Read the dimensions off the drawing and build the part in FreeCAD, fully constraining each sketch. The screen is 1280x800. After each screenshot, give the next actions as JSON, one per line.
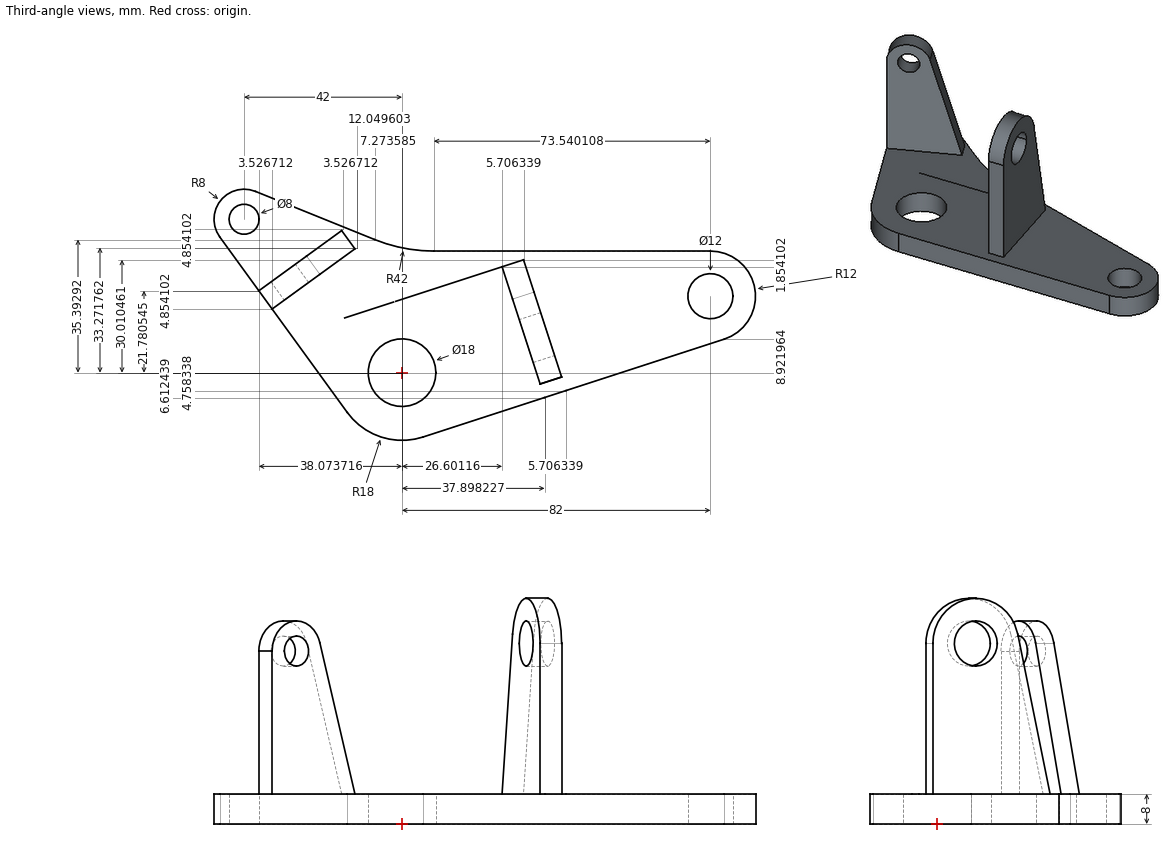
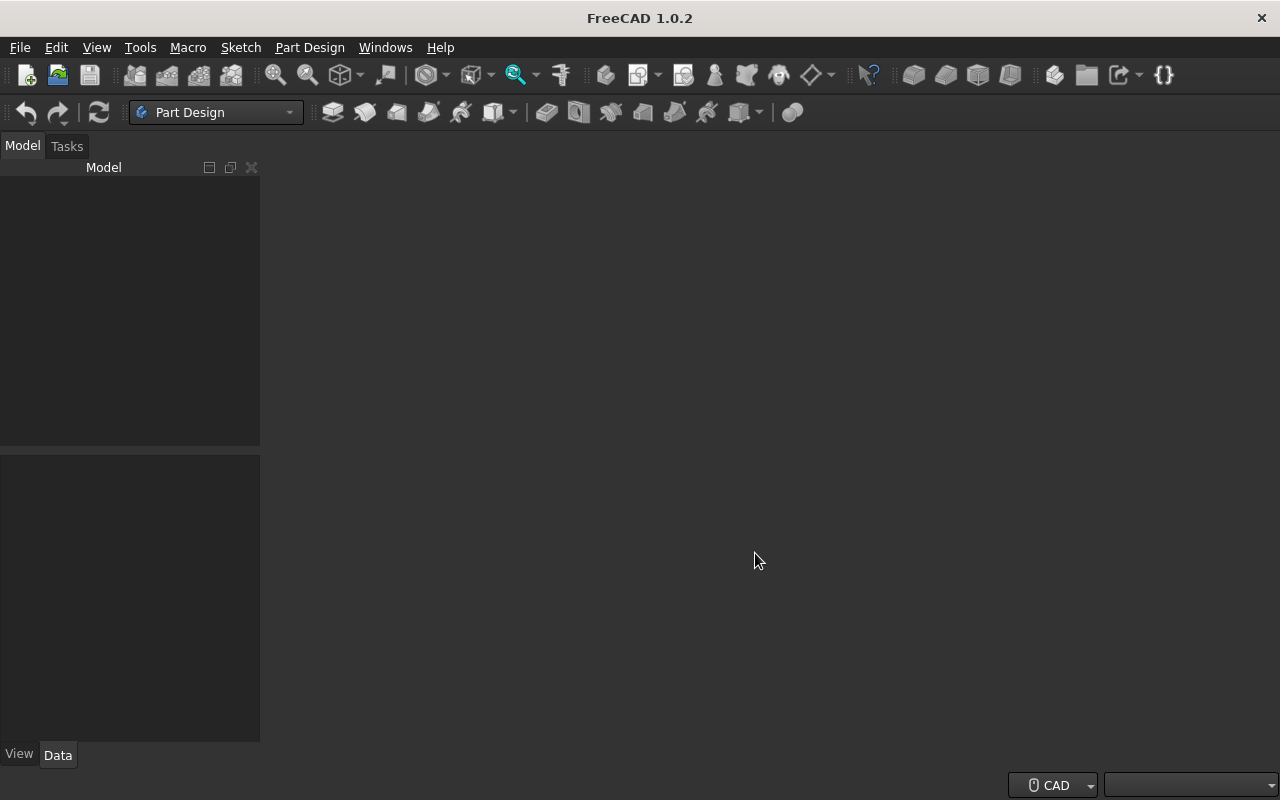
{"action": "left_click", "coordinate": [26, 76]}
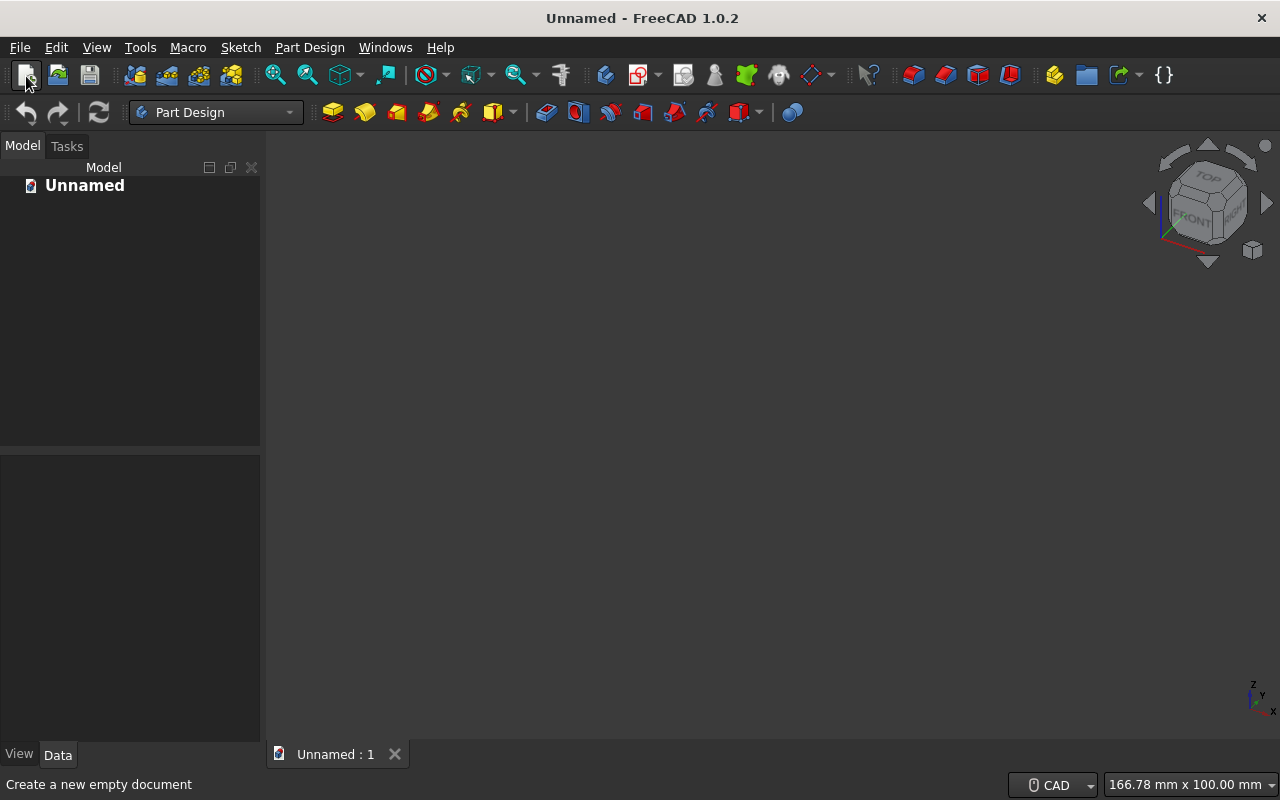
{"action": "left_click", "coordinate": [638, 76]}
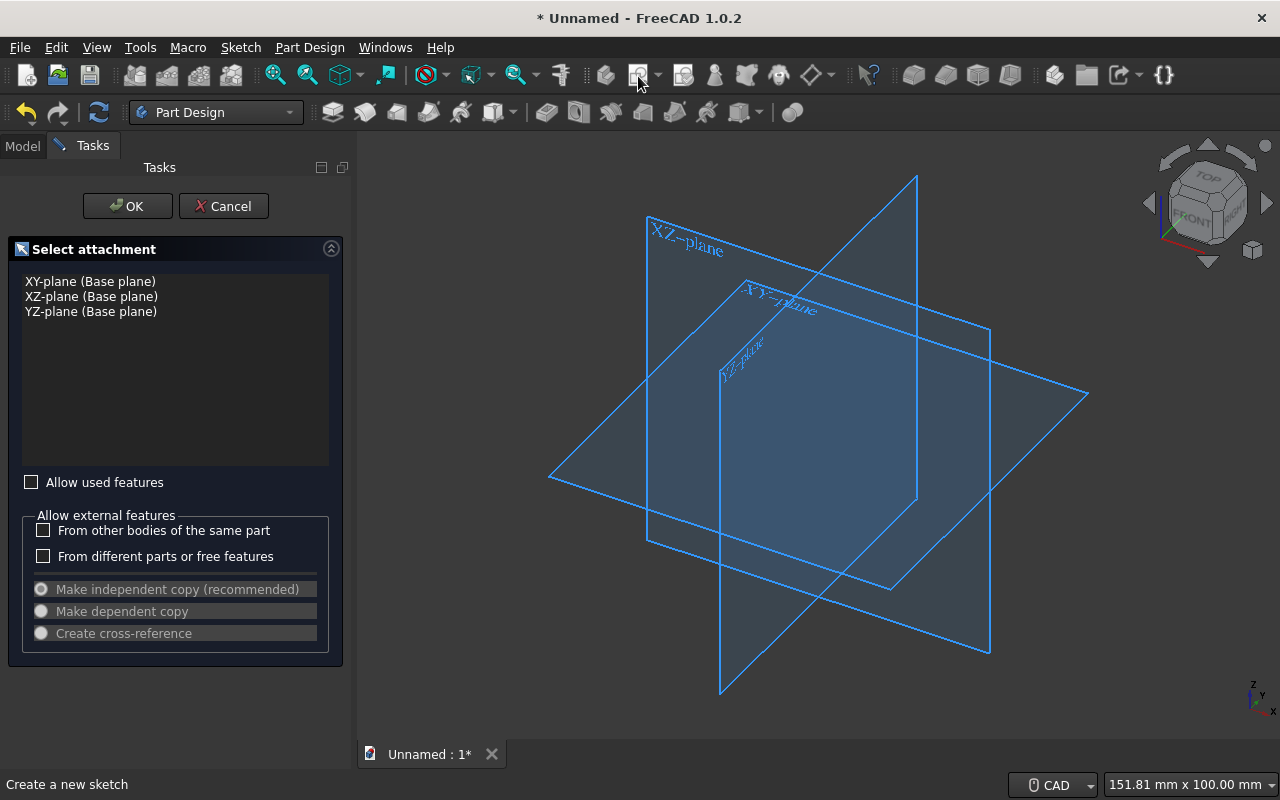
{"action": "left_click", "coordinate": [82, 282]}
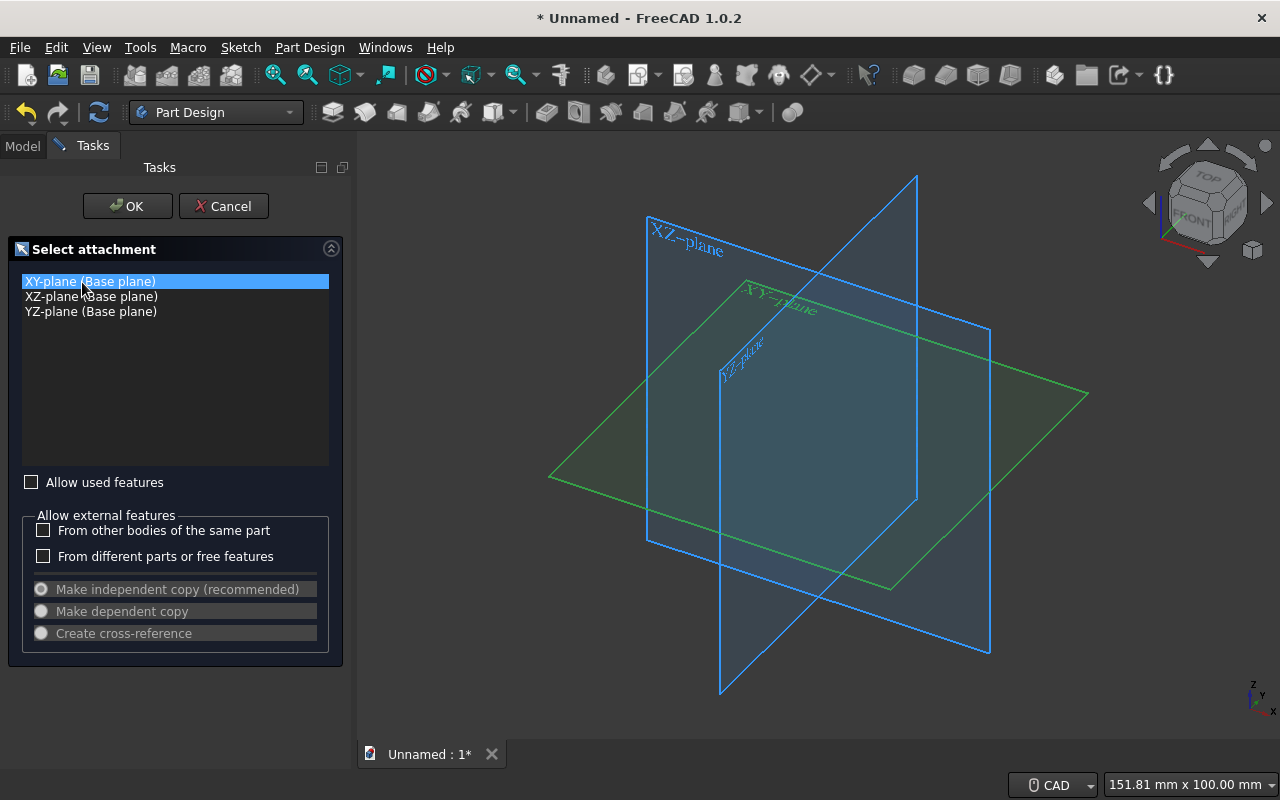
{"action": "left_click", "coordinate": [128, 206]}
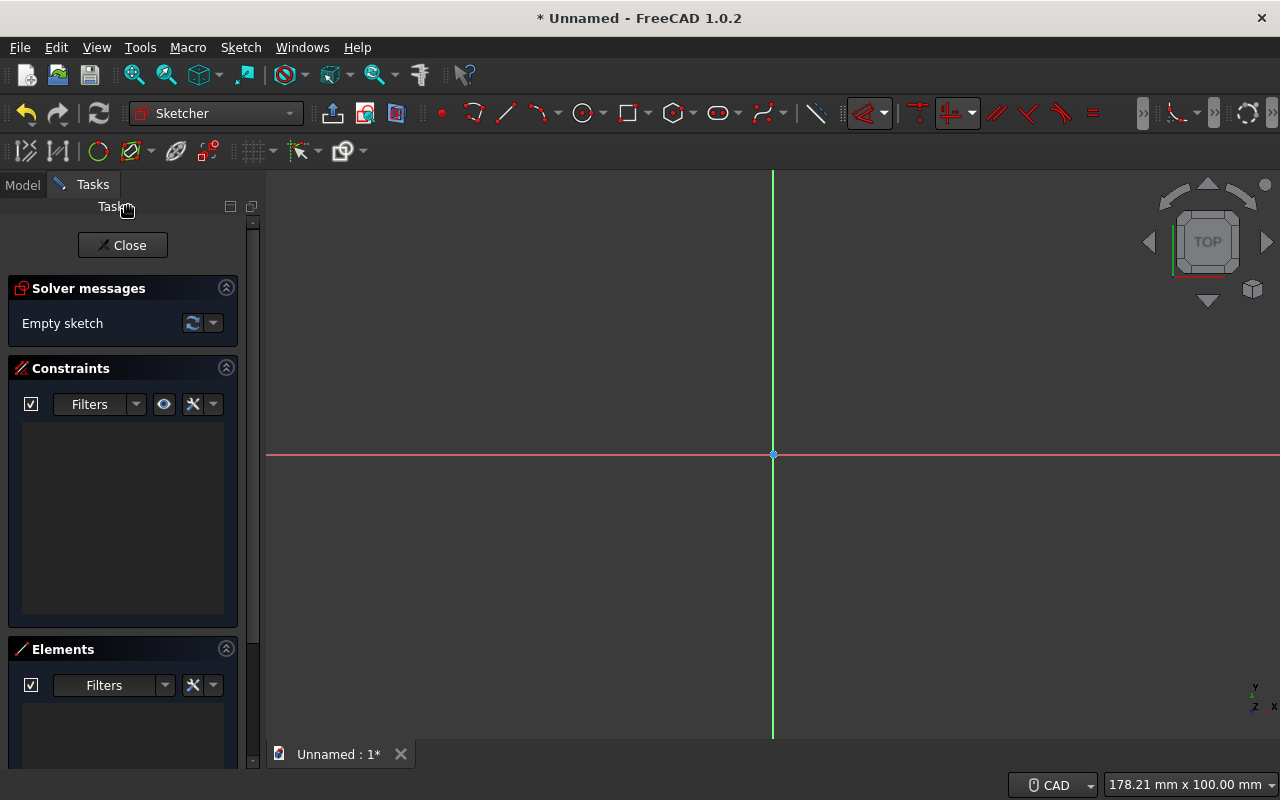
{"action": "scroll", "coordinate": [303, 634], "scroll_direction": "down", "scroll_amount": 2}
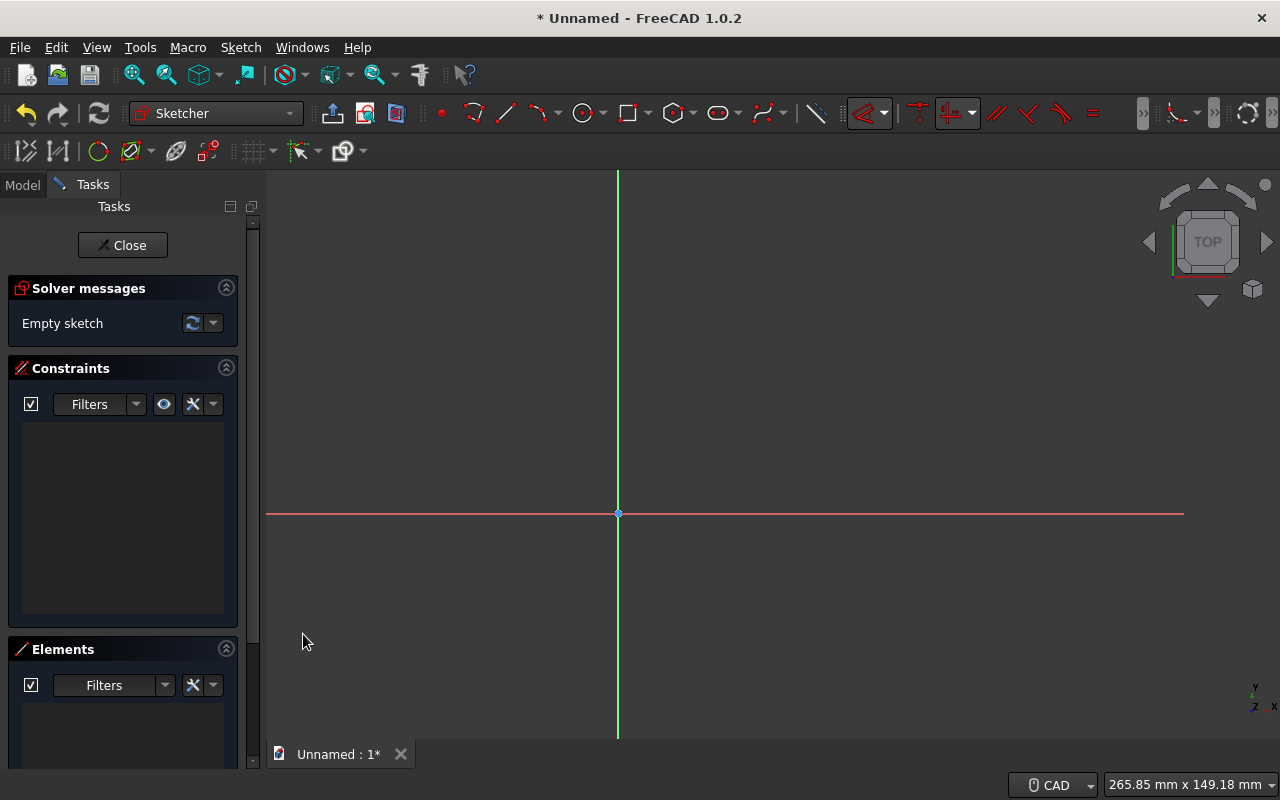
{"action": "key", "text": "g l"}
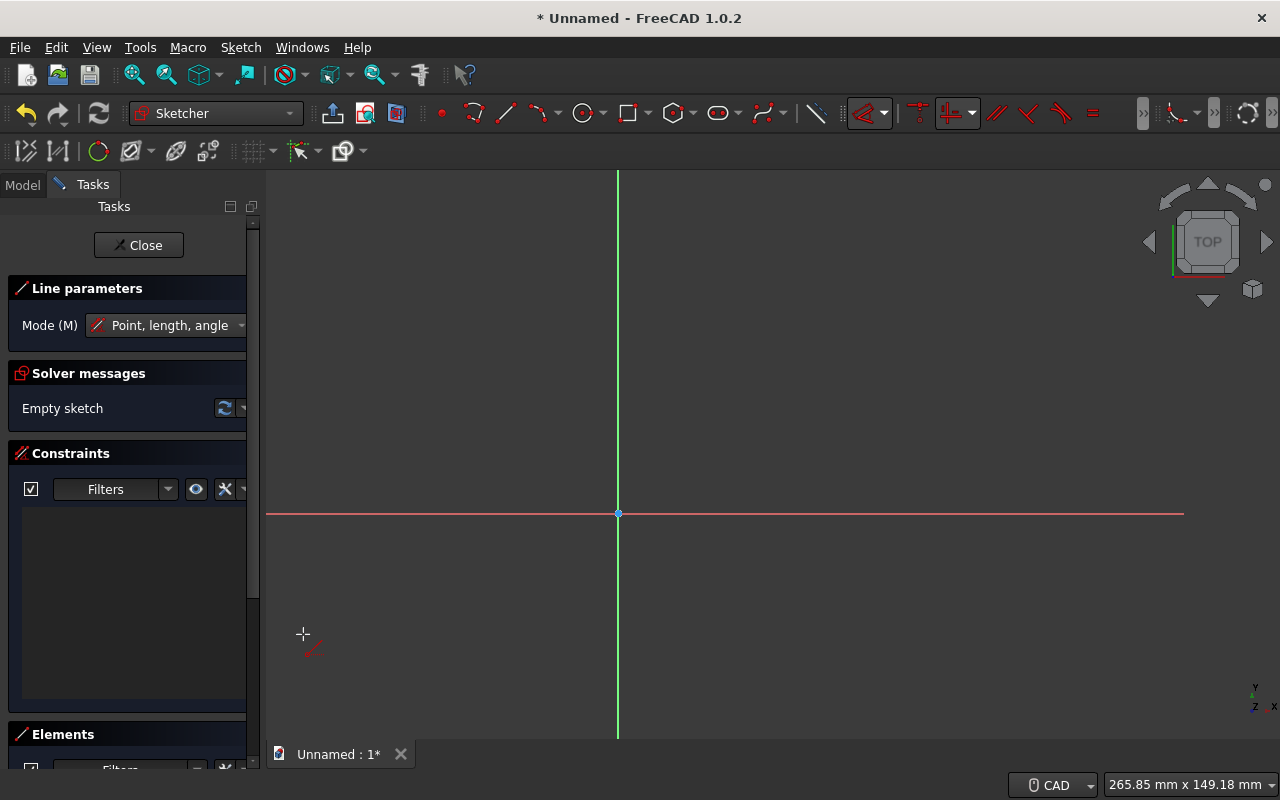
{"action": "left_click", "coordinate": [433, 376]}
{"action": "left_click", "coordinate": [563, 554]}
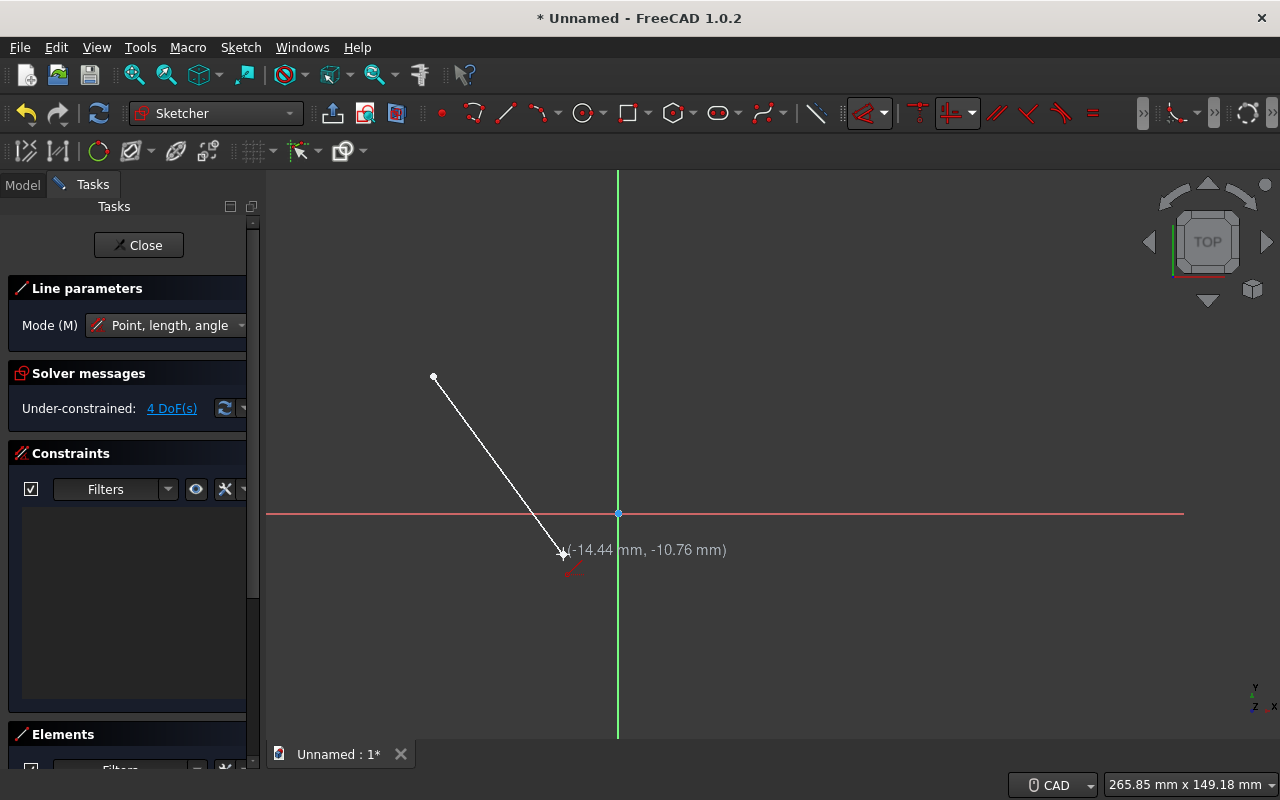
{"action": "left_click", "coordinate": [639, 579]}
{"action": "left_click", "coordinate": [945, 480]}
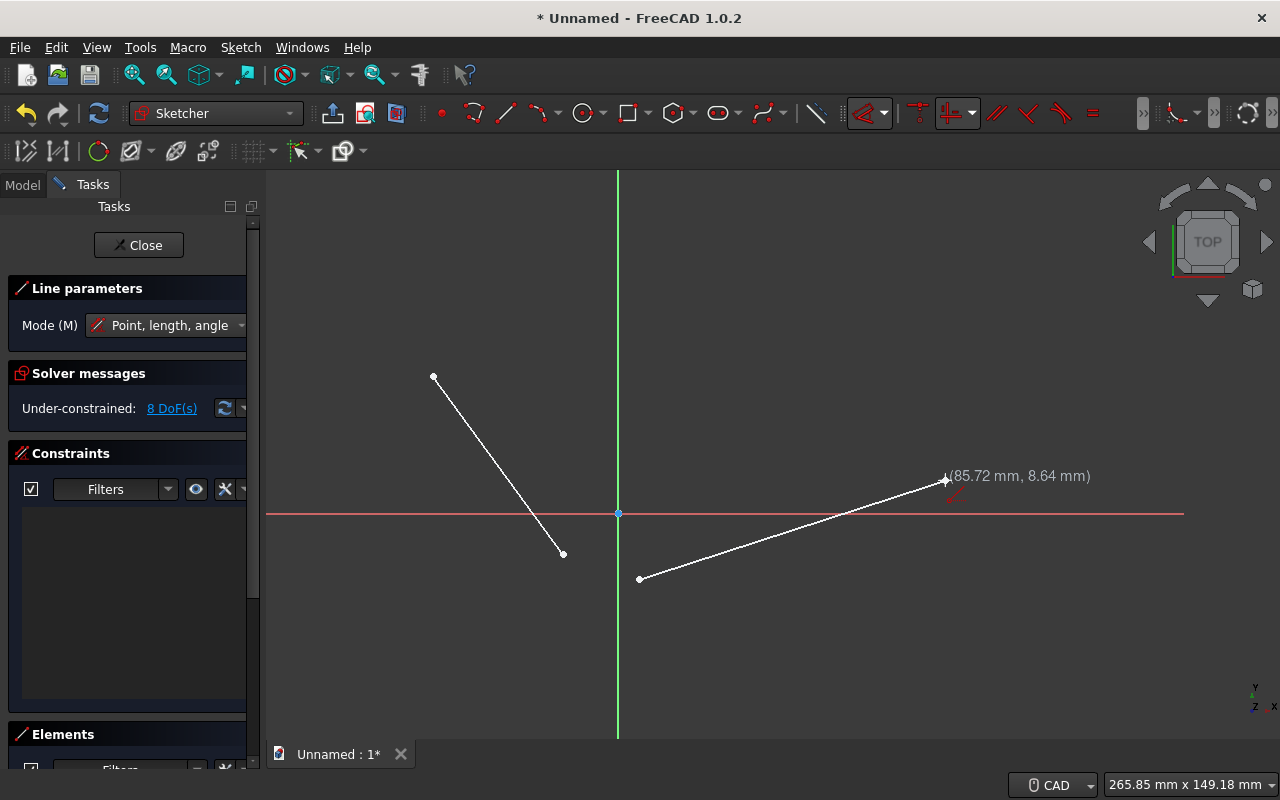
{"action": "left_click", "coordinate": [931, 391]}
{"action": "left_click", "coordinate": [650, 391]}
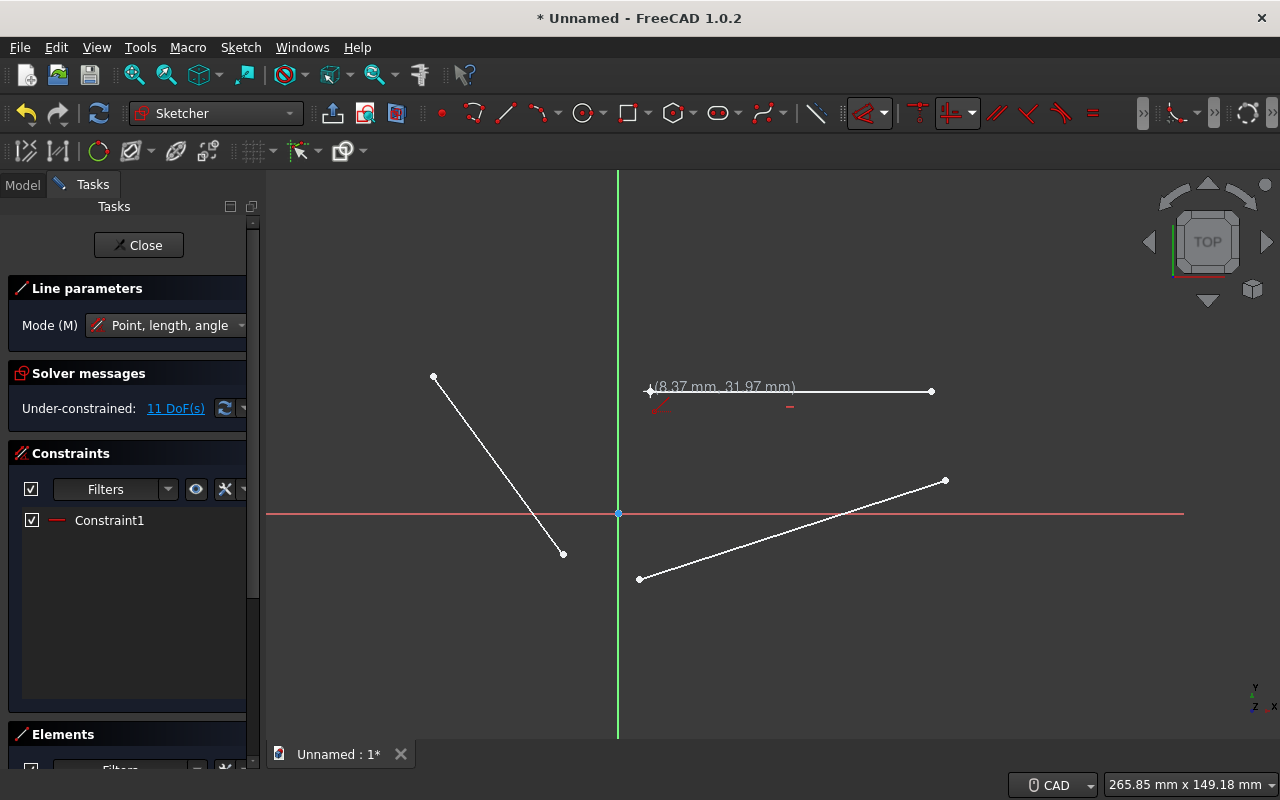
{"action": "left_click", "coordinate": [590, 379]}
{"action": "left_click", "coordinate": [469, 330]}